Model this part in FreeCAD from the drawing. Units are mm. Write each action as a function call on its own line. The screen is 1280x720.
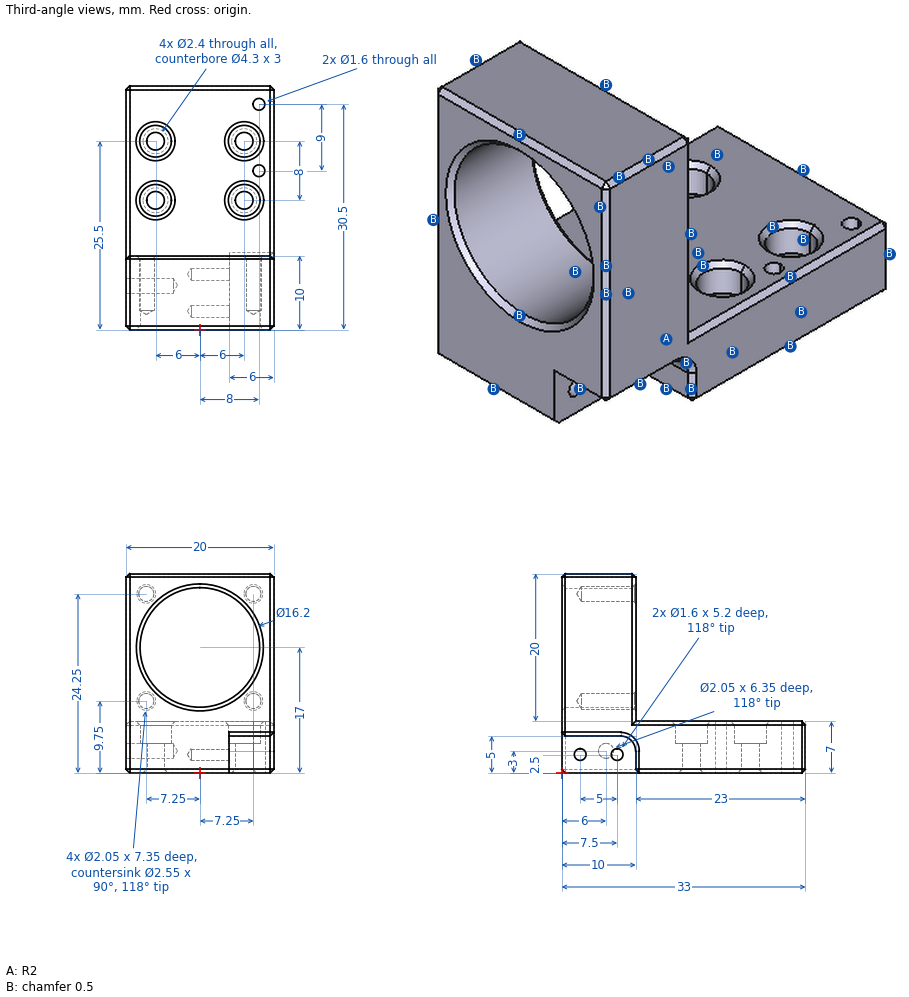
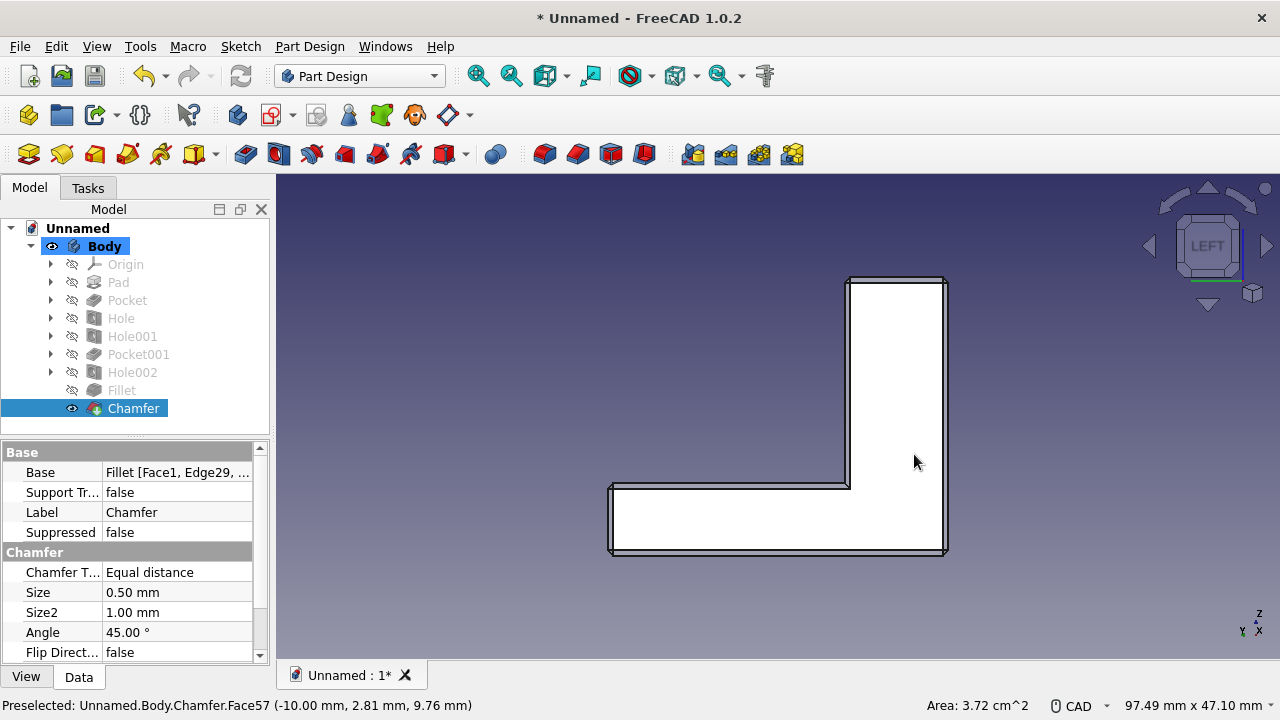
click(270, 116)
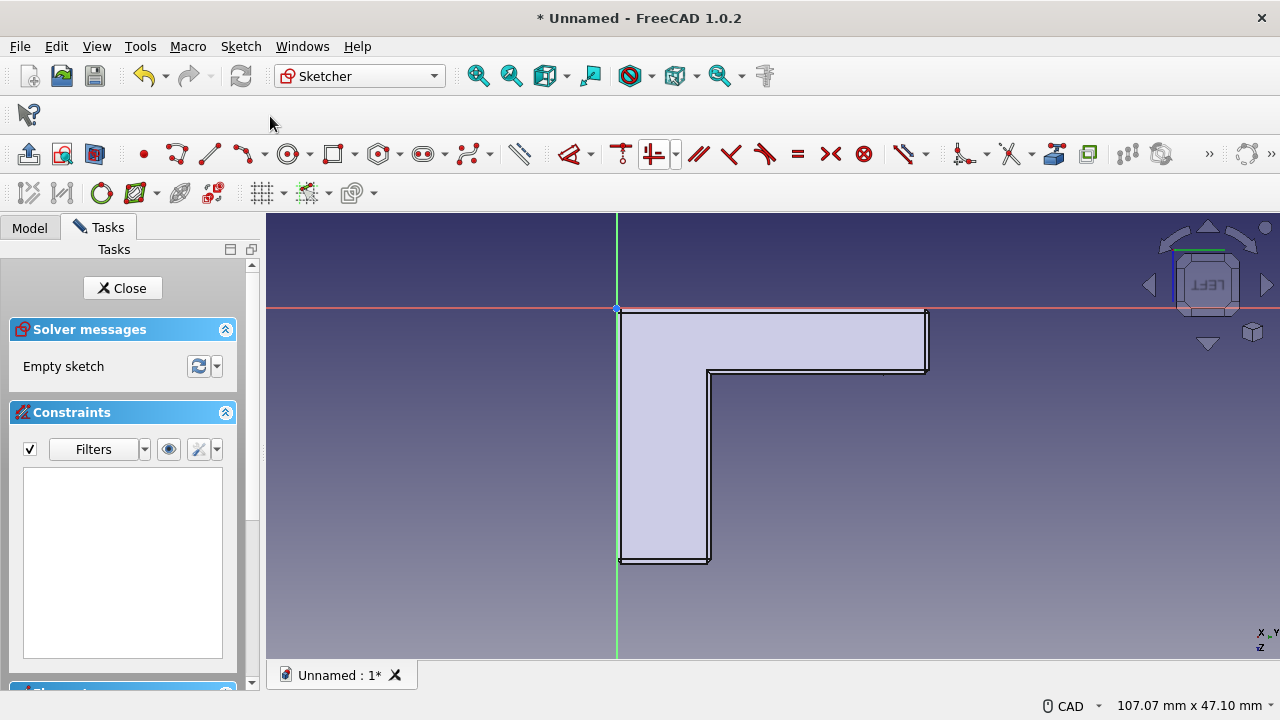
scroll(671, 329, up, 13)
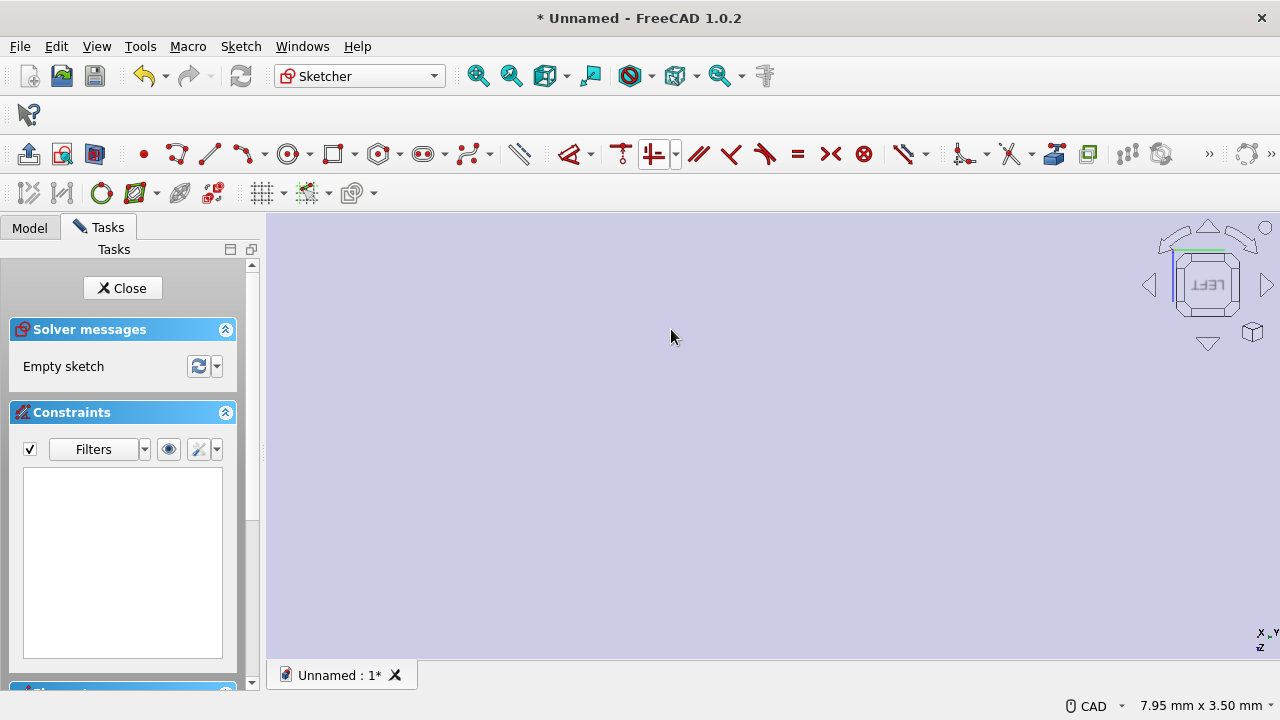
key(g)
key(c)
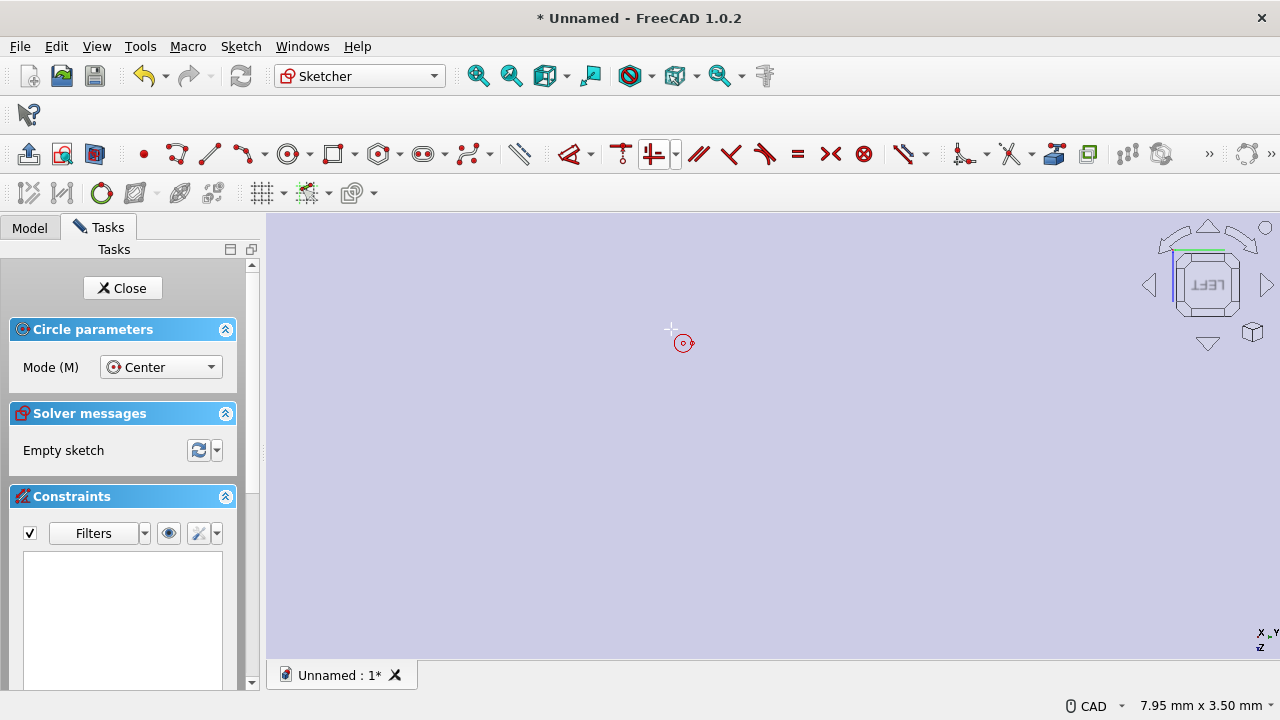
click(701, 428)
move(793, 335)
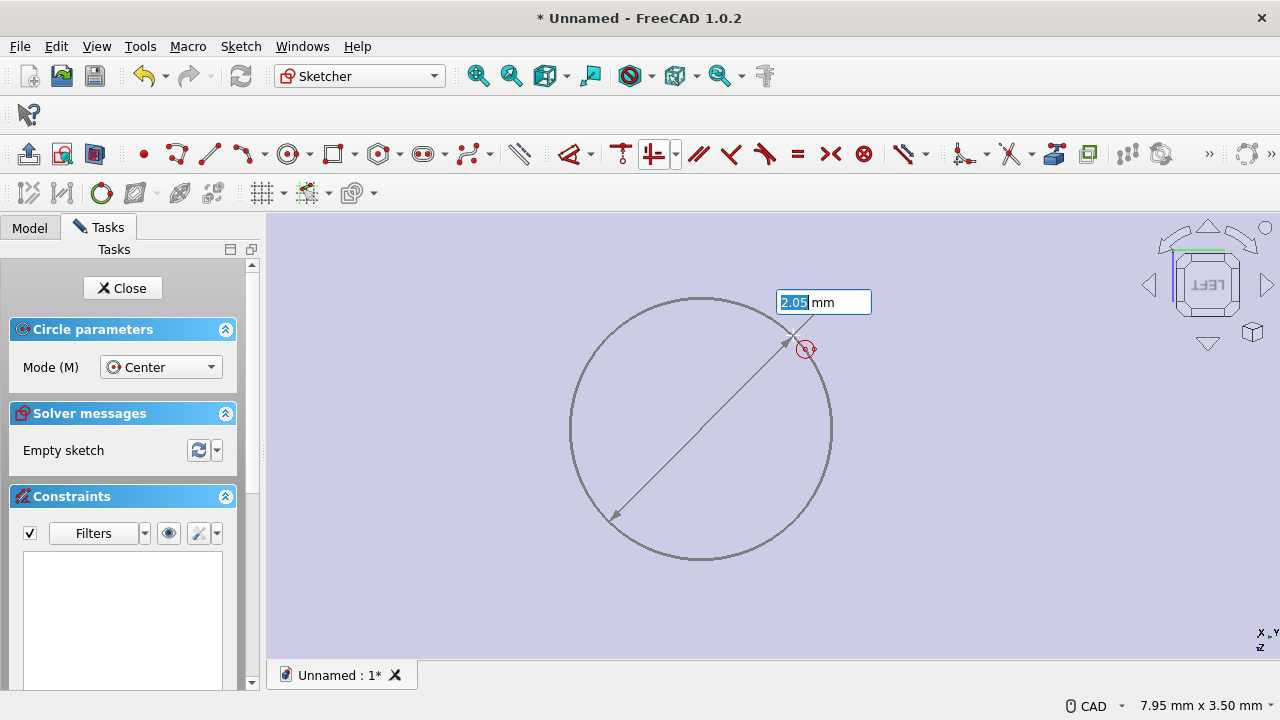
text(2.05)
key(Return)
key(Escape)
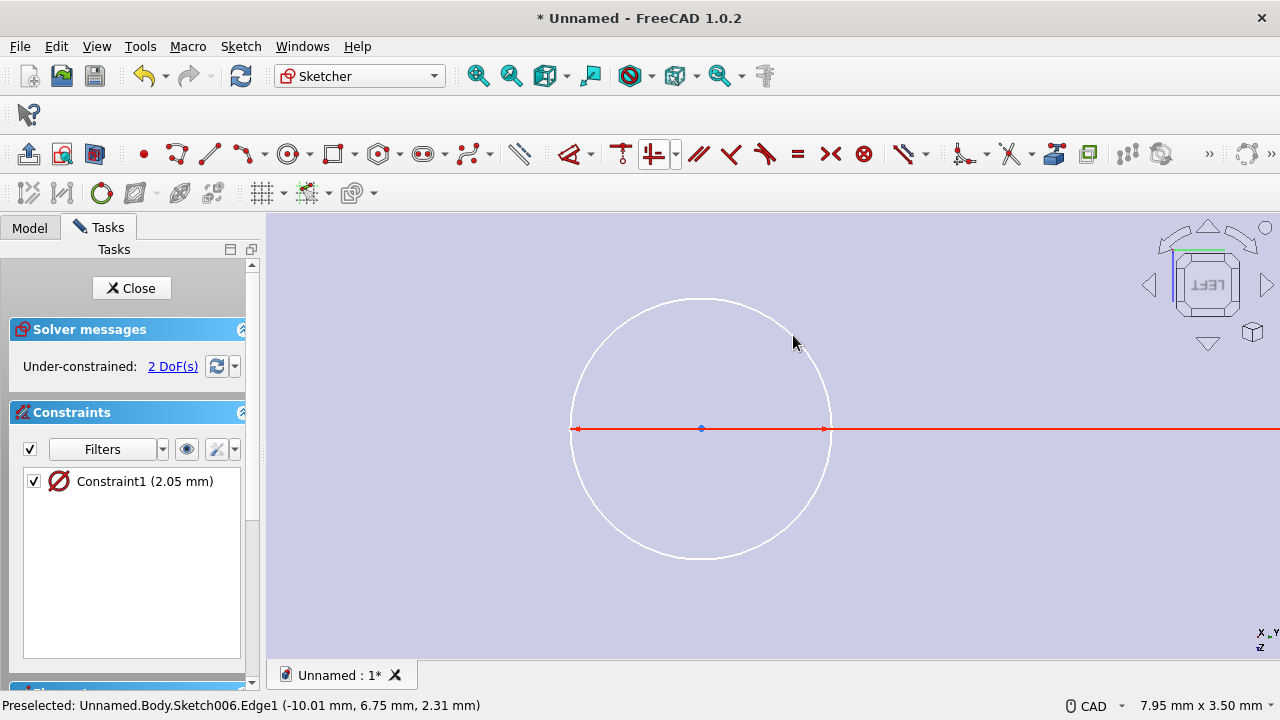
key(d)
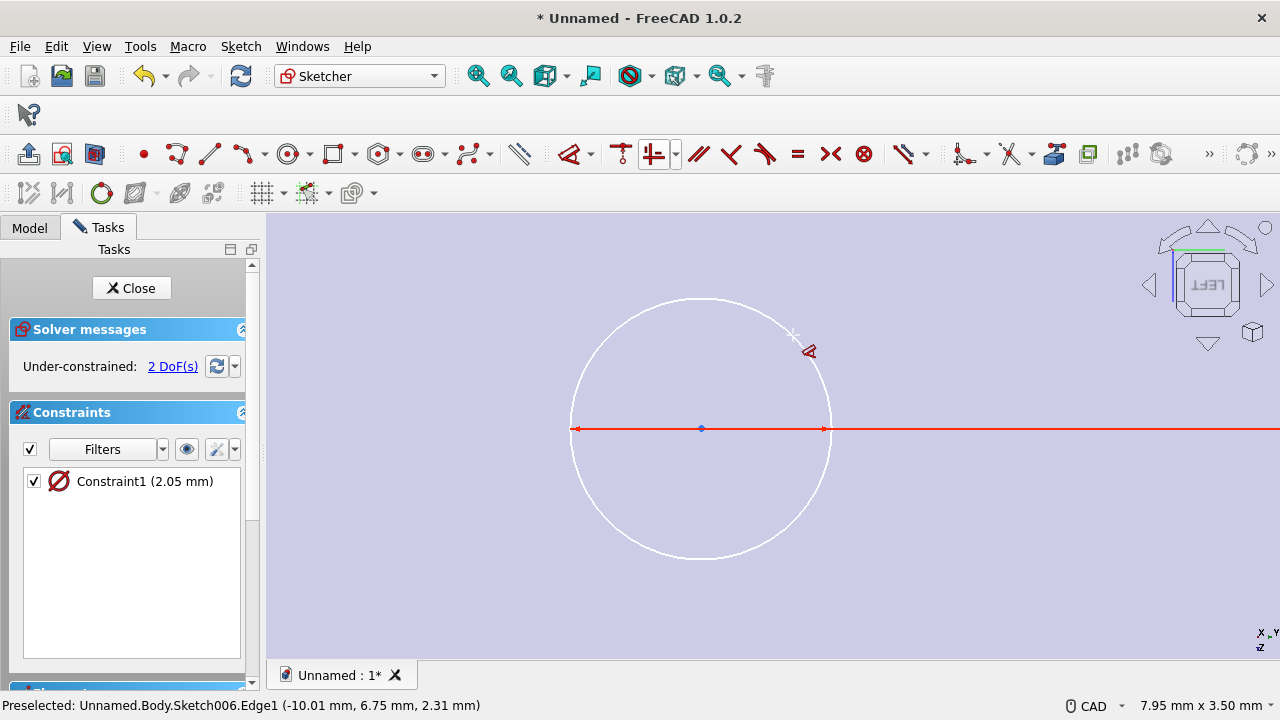
click(701, 429)
click(498, 463)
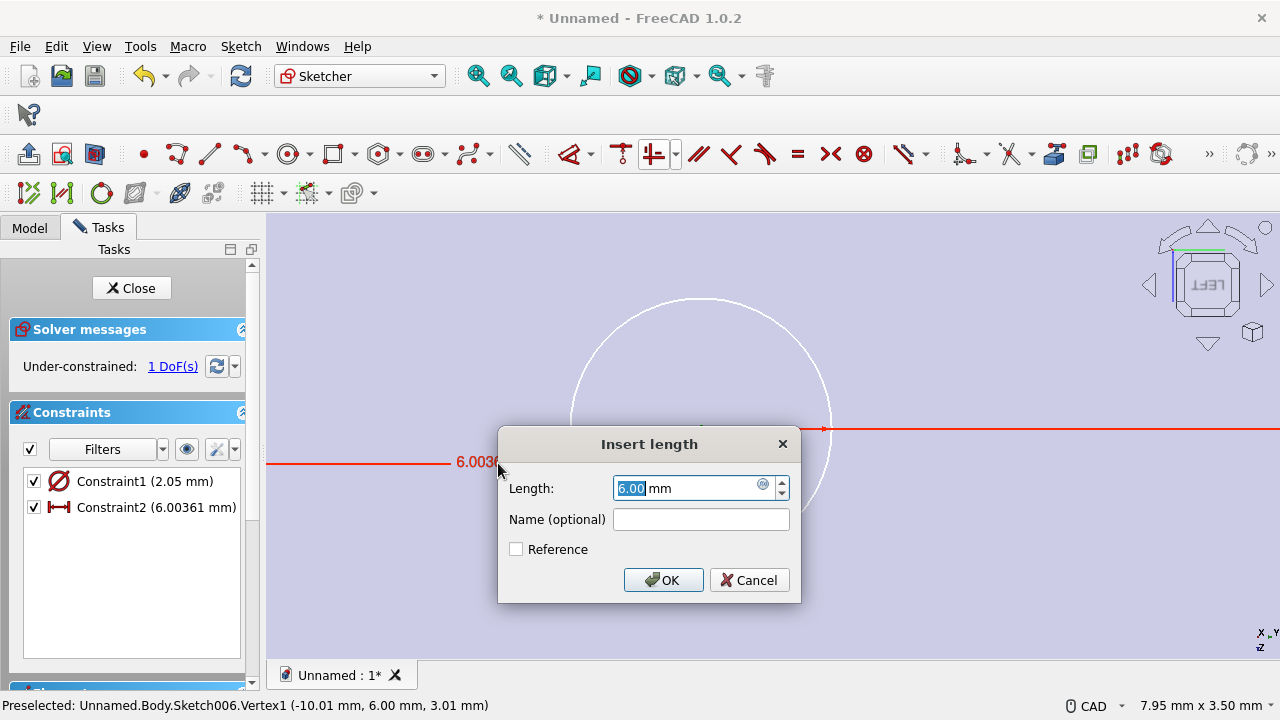
text(6)
key(Return)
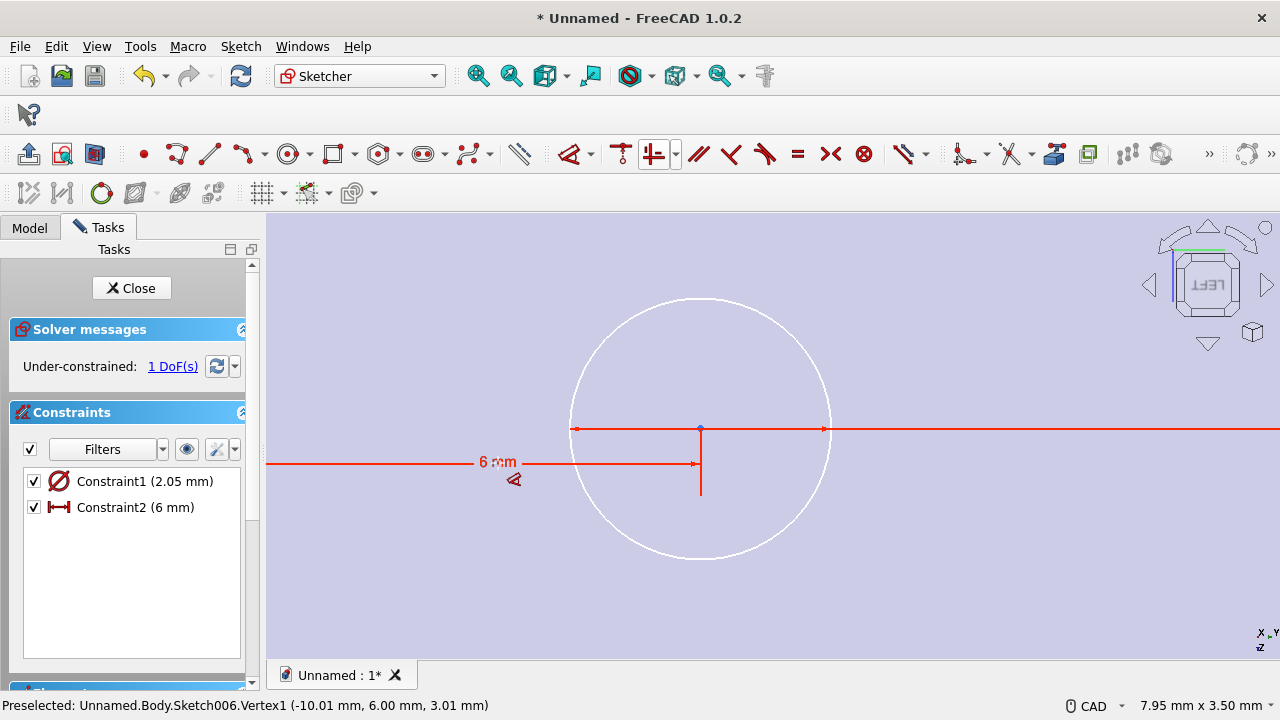
click(701, 429)
click(735, 335)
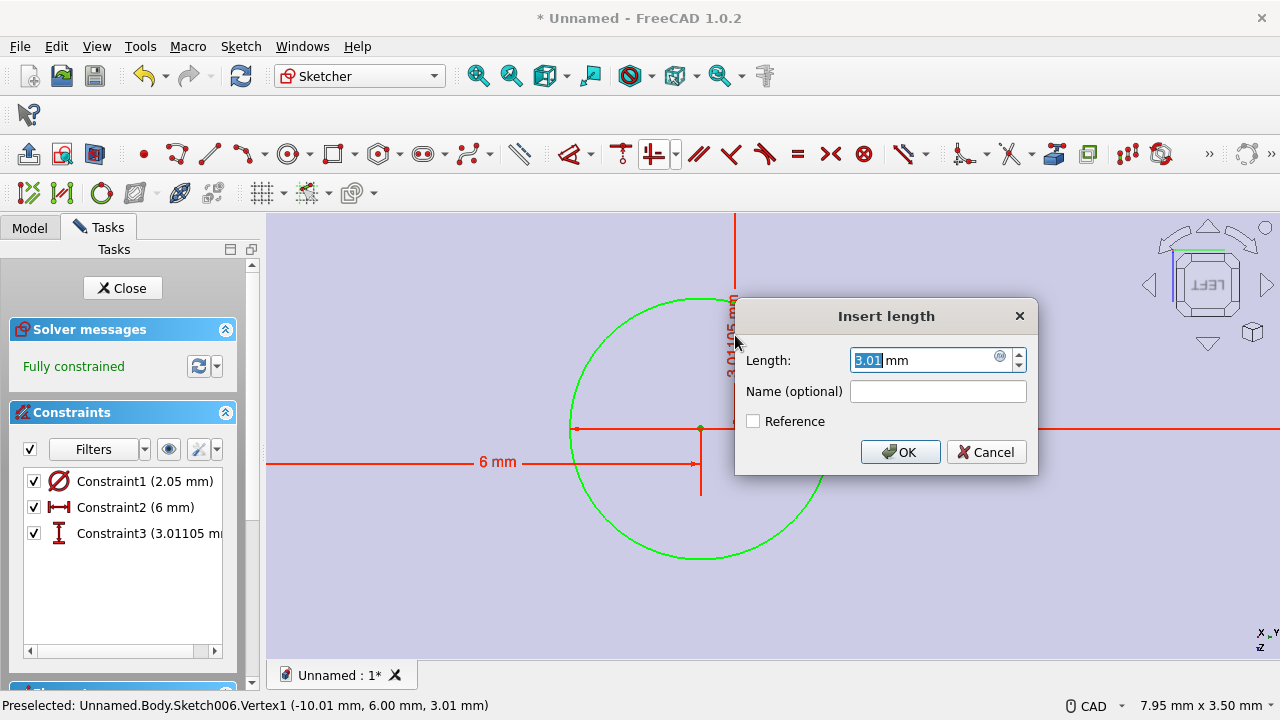
text(3)
key(Return)
key(Escape)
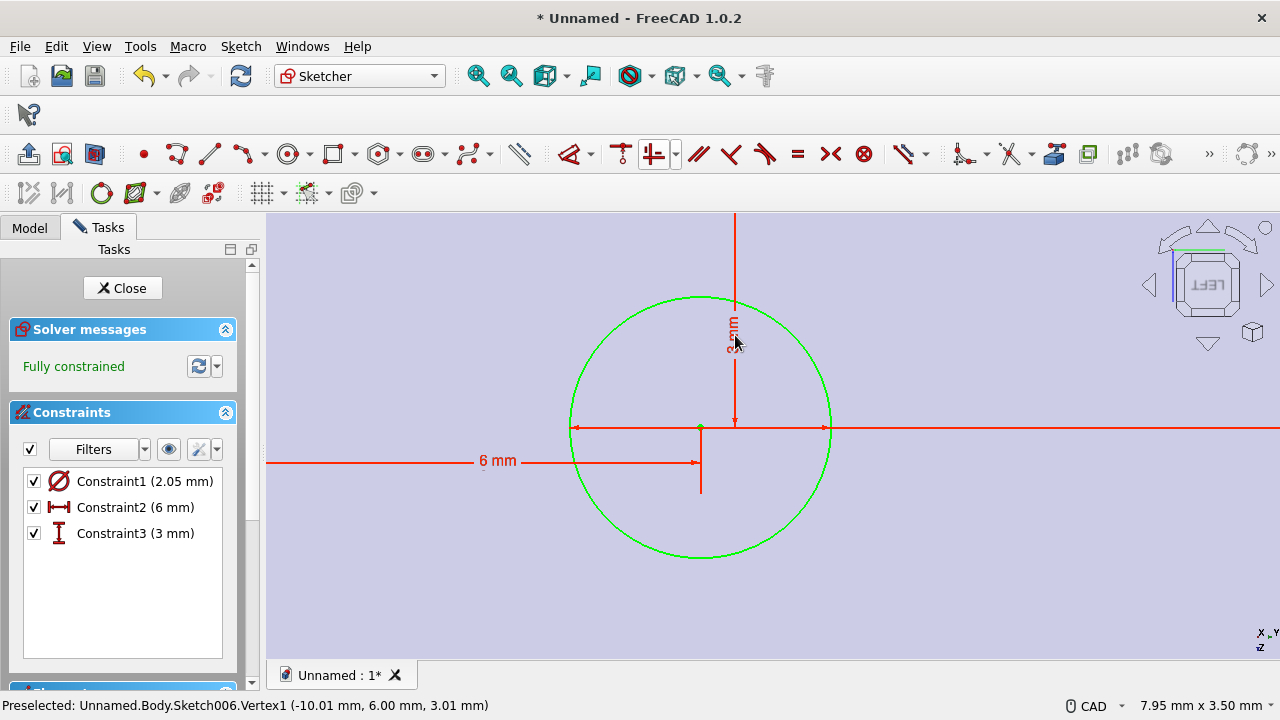
click(123, 288)